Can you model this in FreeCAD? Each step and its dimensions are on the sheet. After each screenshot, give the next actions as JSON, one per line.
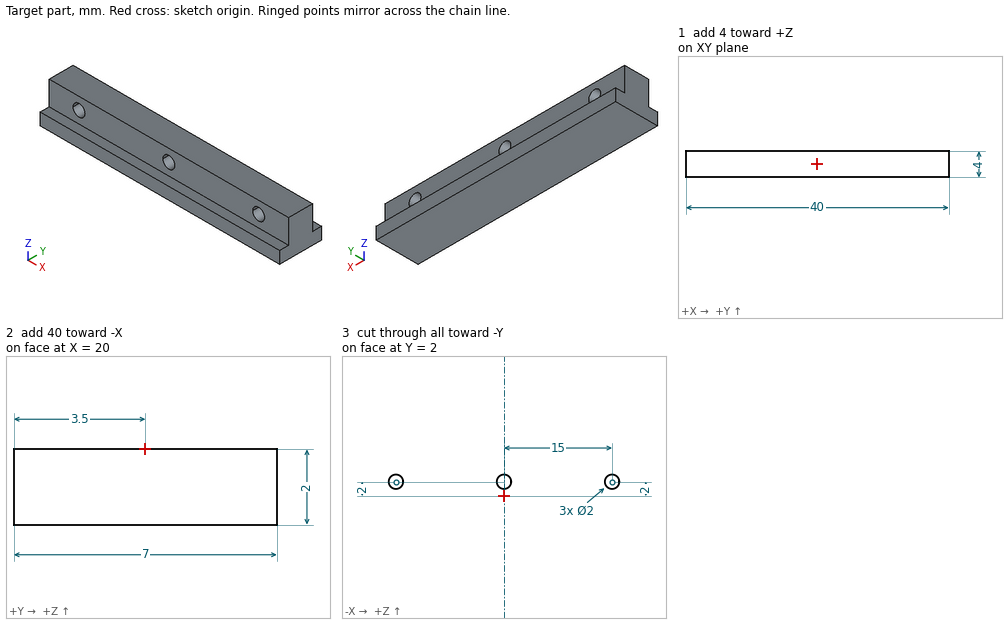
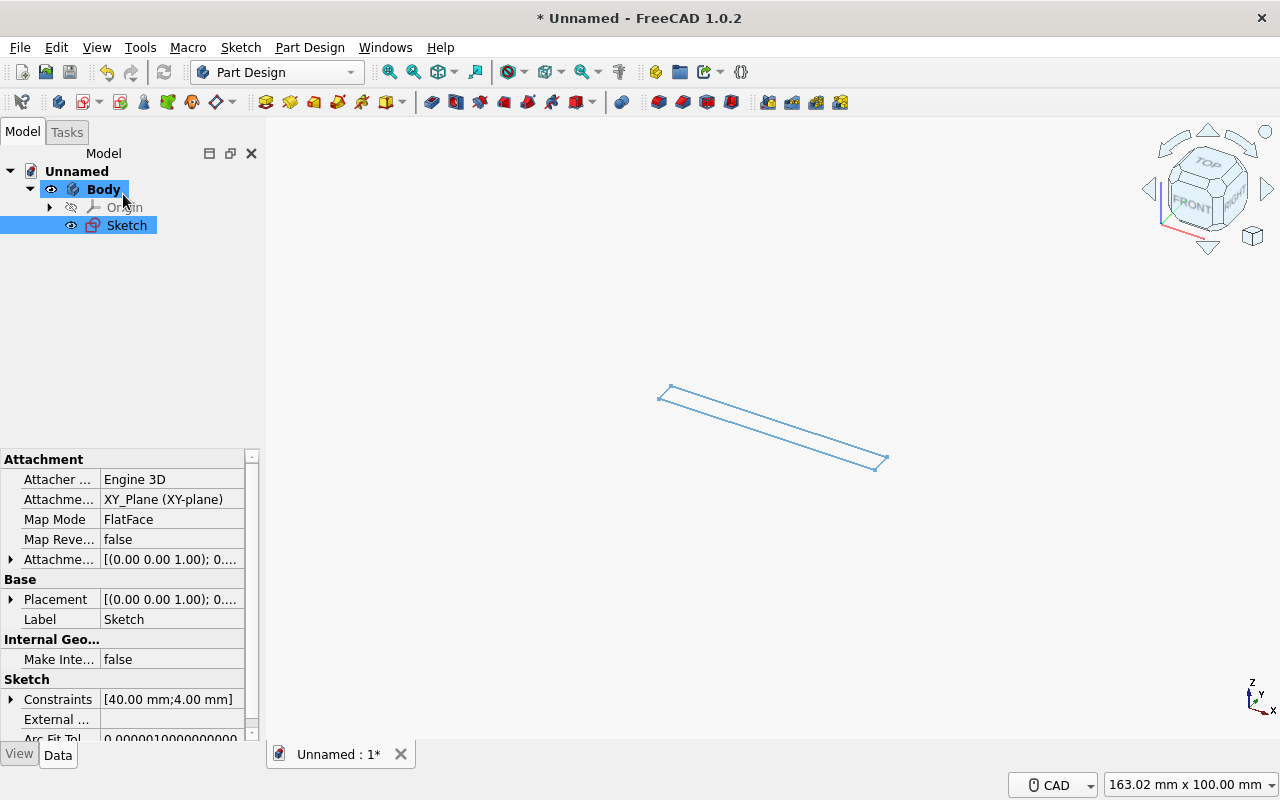
{"action": "left_click", "coordinate": [266, 102]}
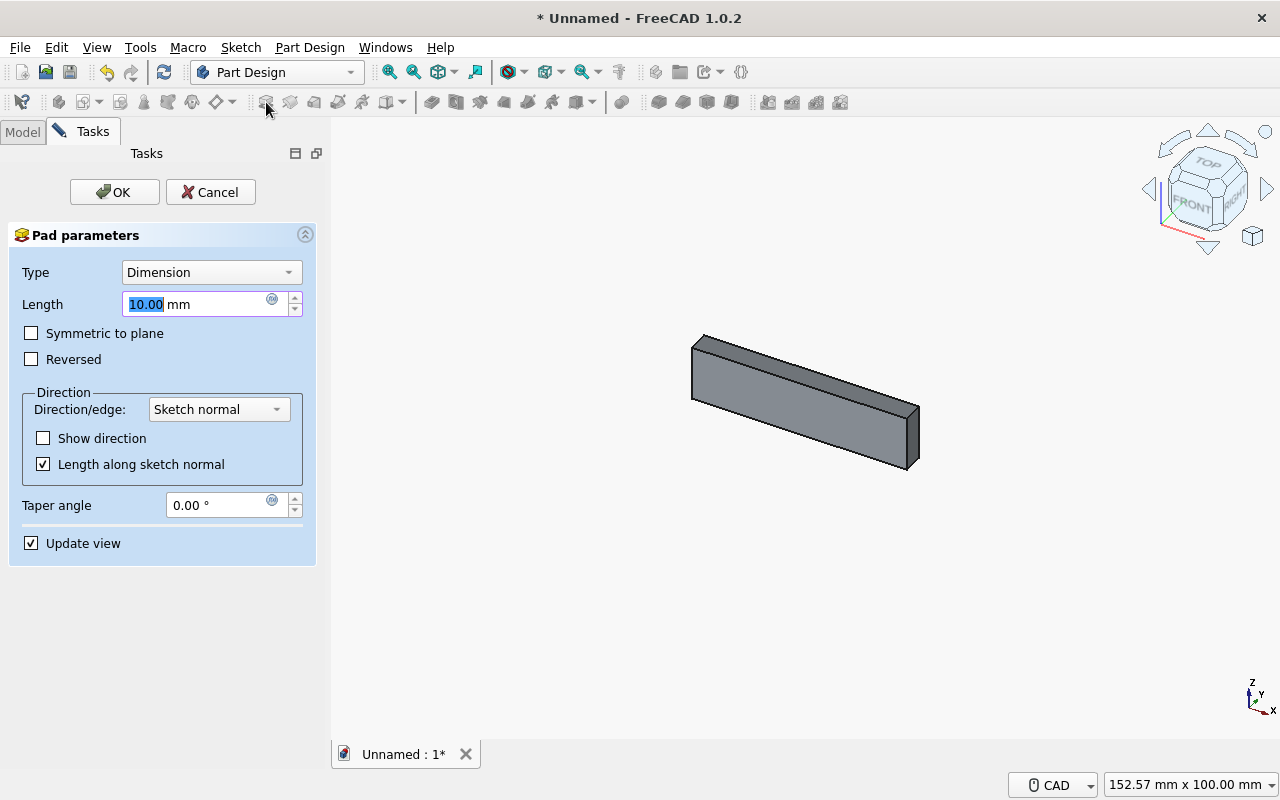
{"action": "type", "text": "4"}
{"action": "key", "text": "Tab"}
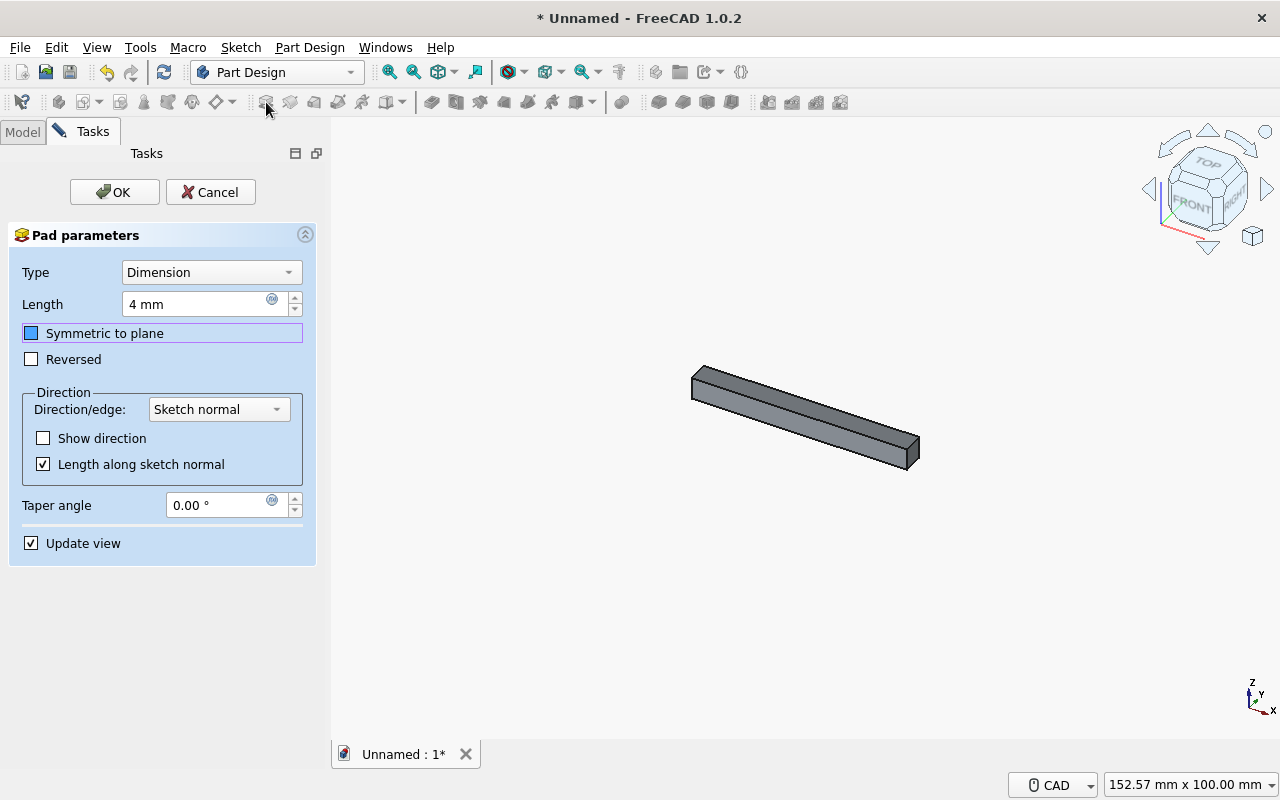
{"action": "left_click", "coordinate": [115, 192]}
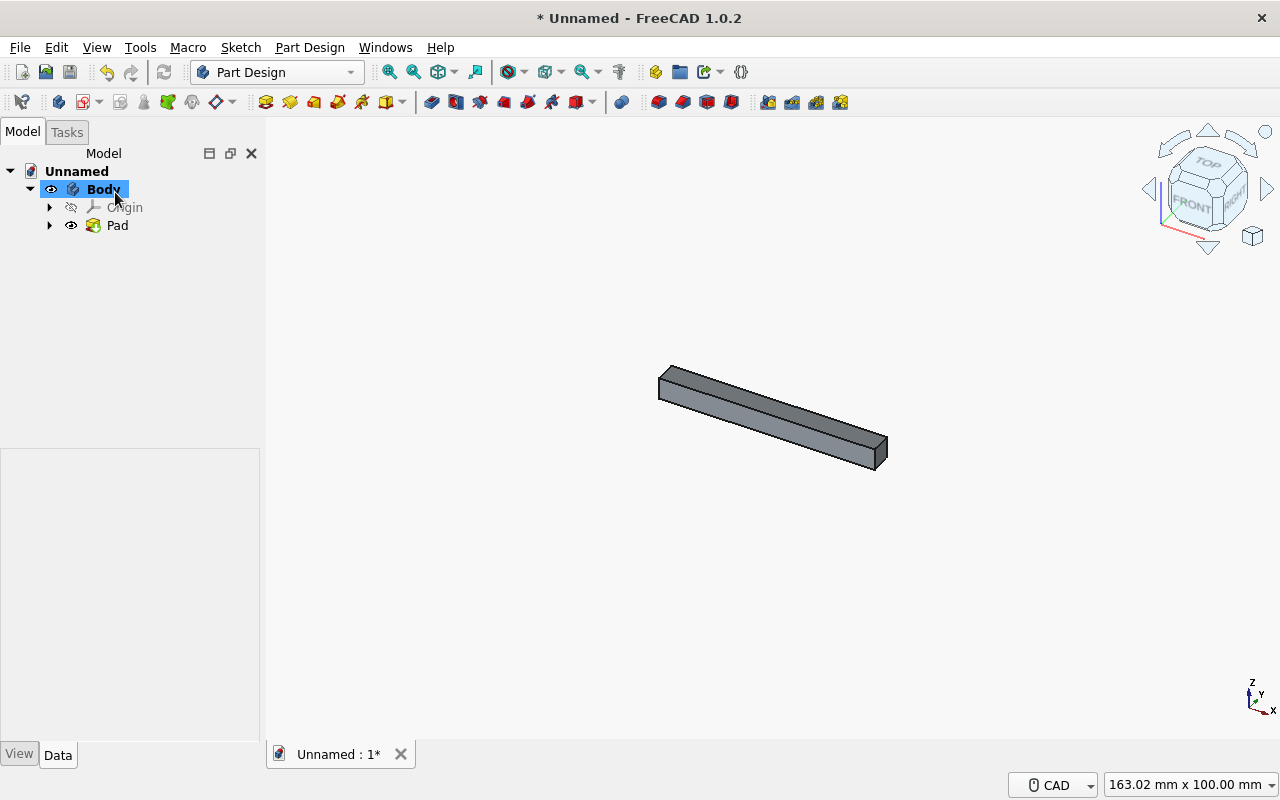
{"action": "key", "text": "v f"}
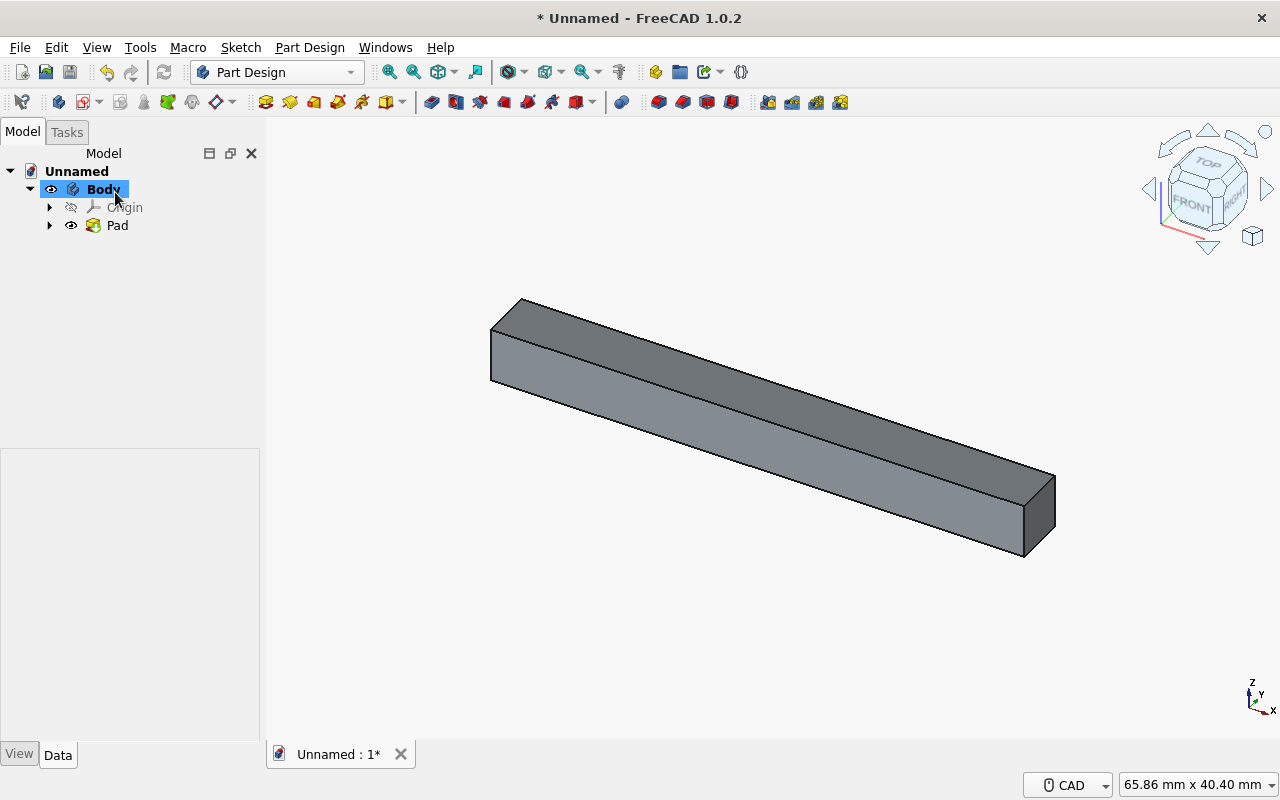
{"action": "left_click", "coordinate": [1040, 515]}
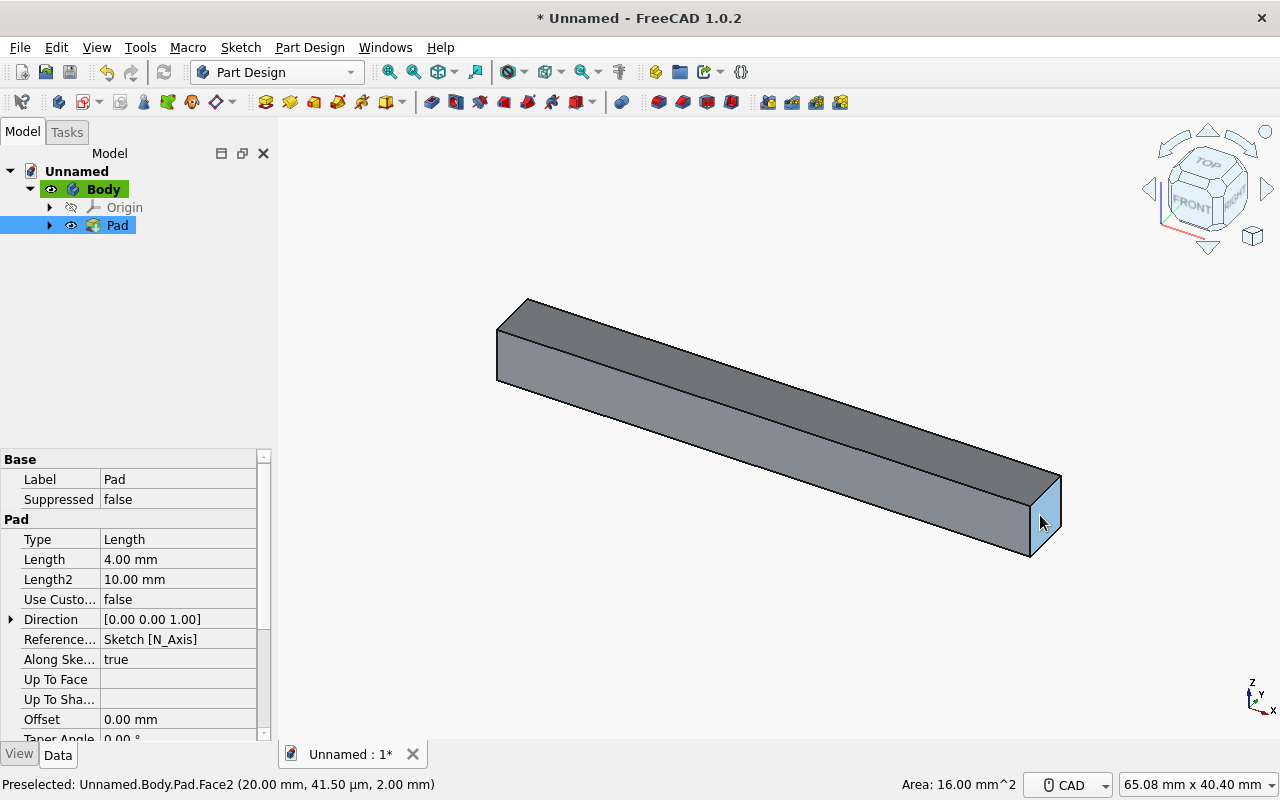
{"action": "left_click", "coordinate": [84, 102]}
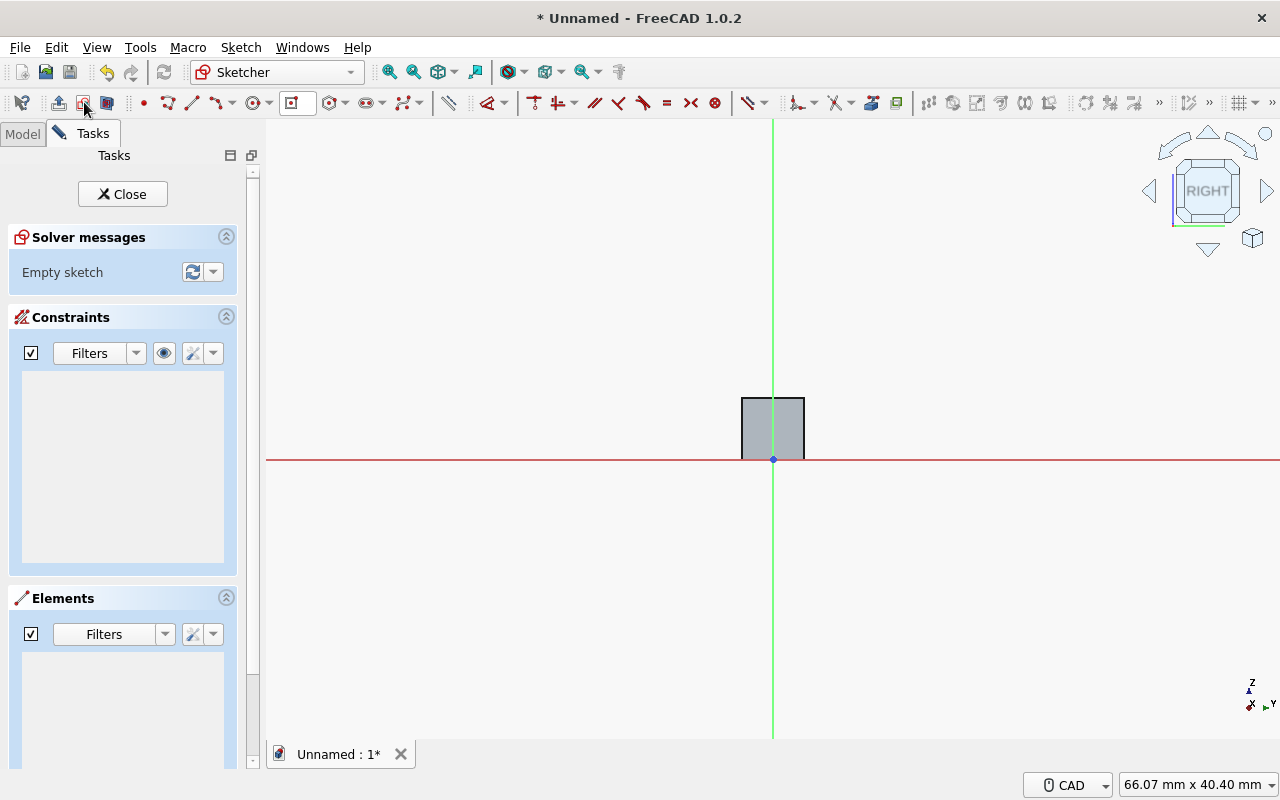
{"action": "scroll", "coordinate": [790, 487], "scroll_direction": "up", "scroll_amount": 8}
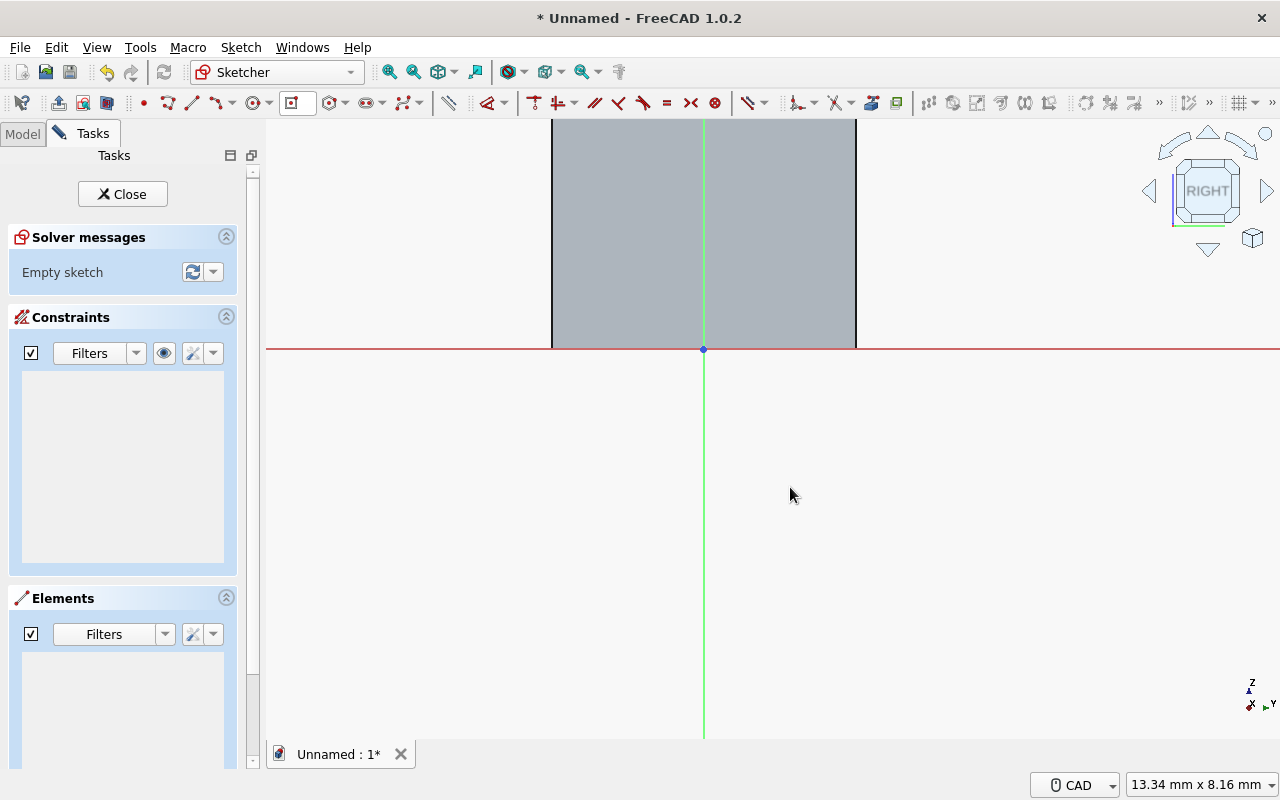
{"action": "key", "text": "g r"}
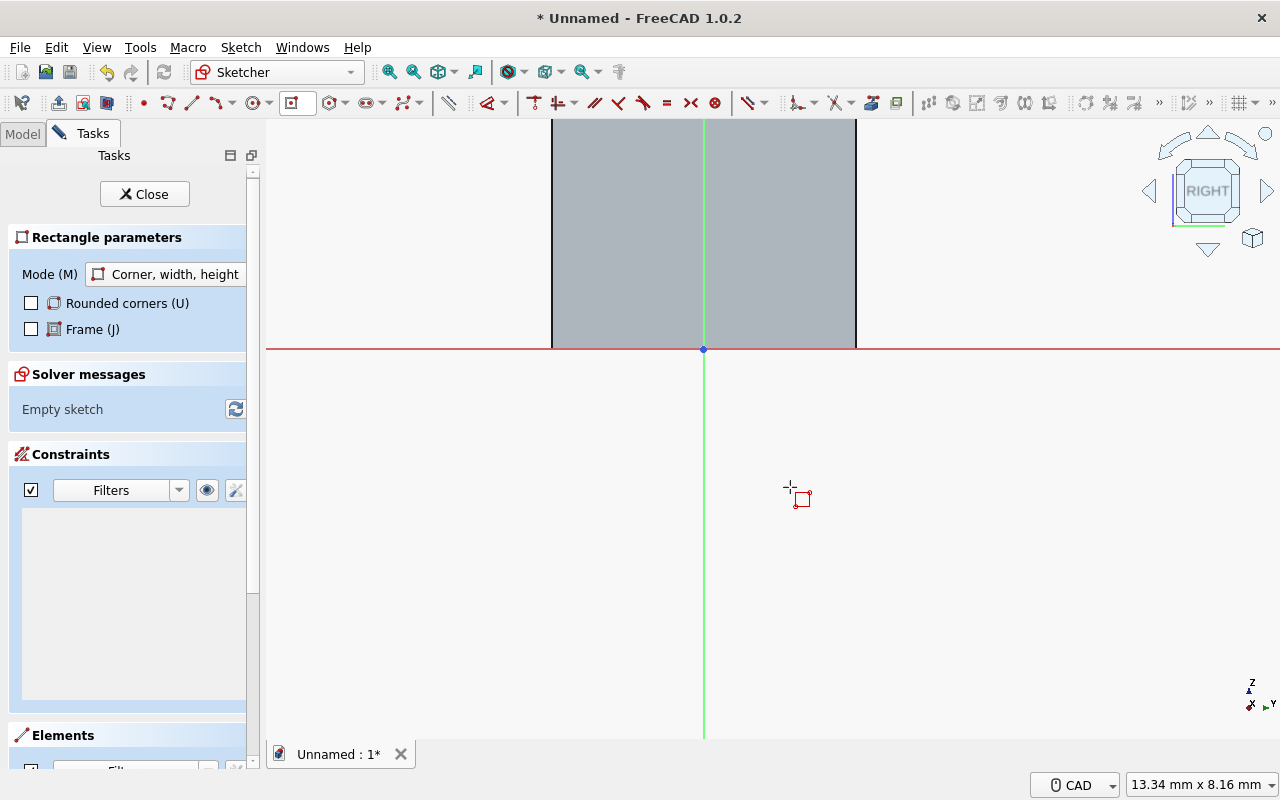
{"action": "left_click", "coordinate": [438, 349]}
{"action": "mouse_move", "coordinate": [970, 501]}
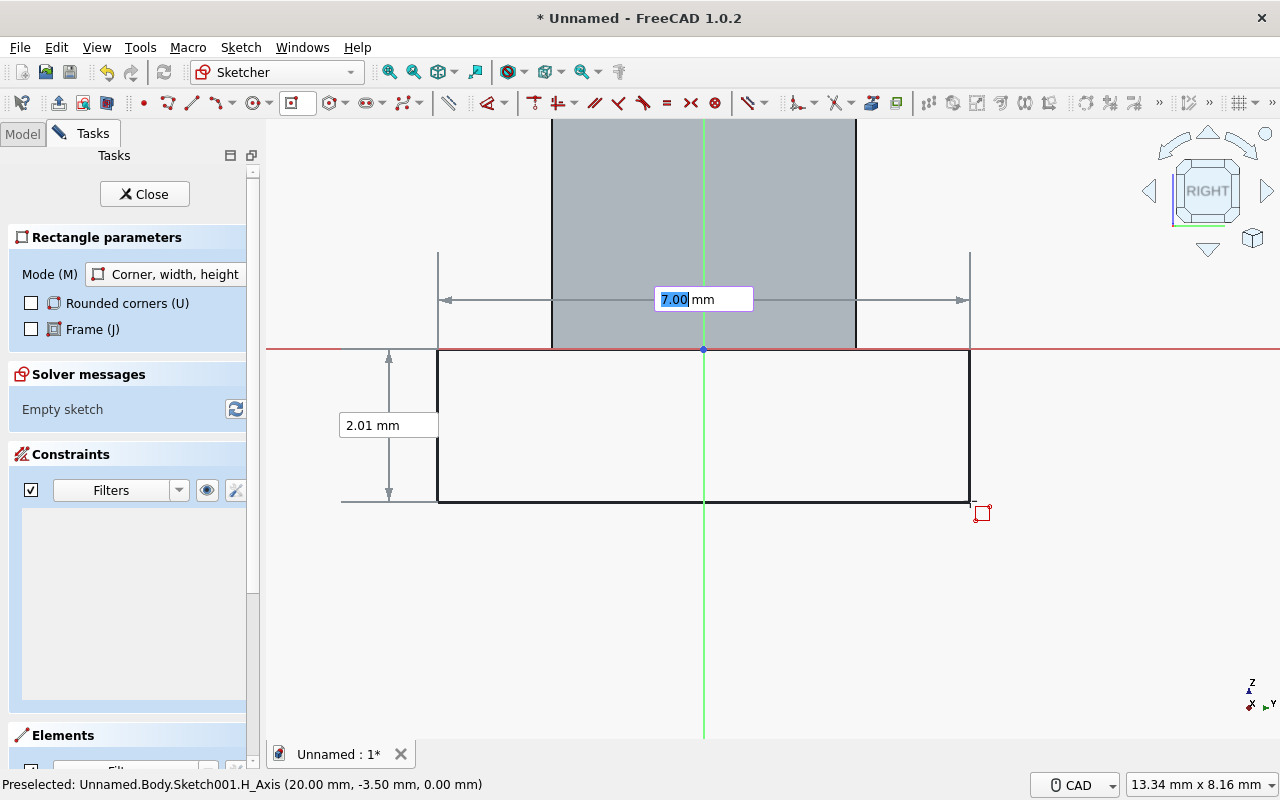
{"action": "type", "text": "7"}
{"action": "key", "text": "Tab"}
{"action": "type", "text": "2"}
{"action": "key", "text": "Return"}
{"action": "key", "text": "Escape"}